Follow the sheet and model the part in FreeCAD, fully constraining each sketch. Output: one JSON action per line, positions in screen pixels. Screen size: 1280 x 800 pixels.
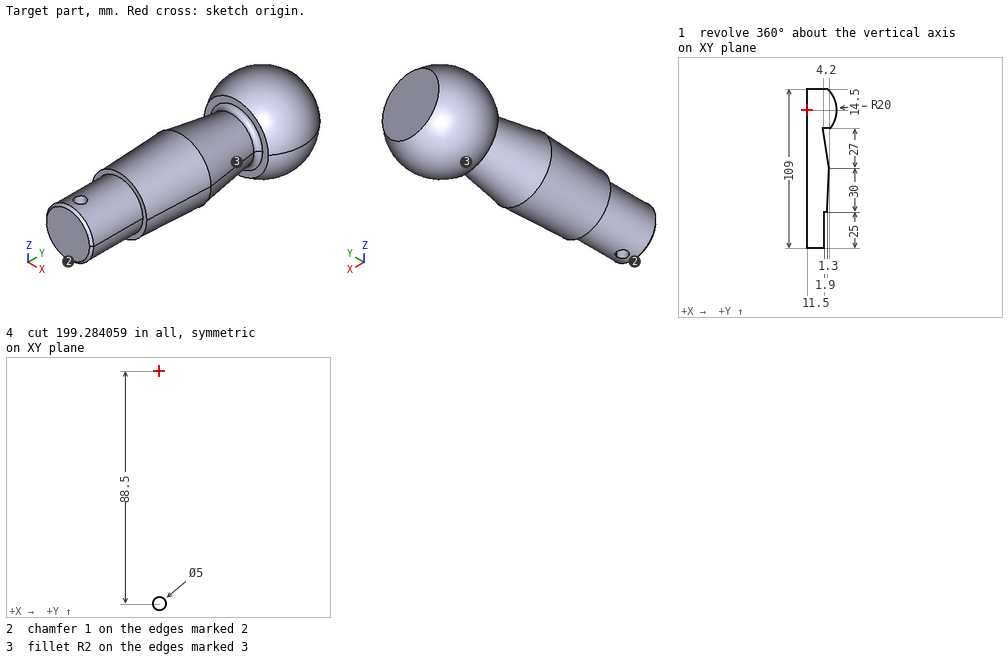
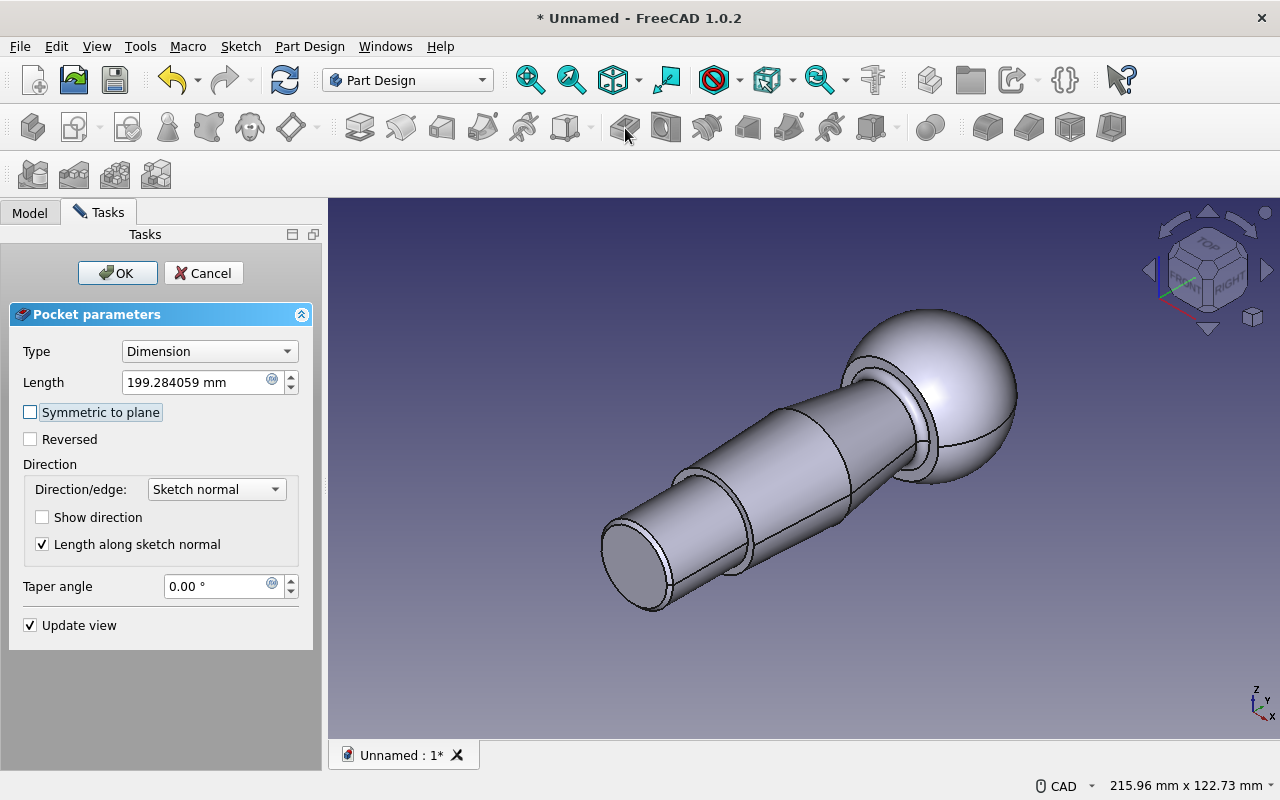
{"action": "left_click", "coordinate": [31, 412]}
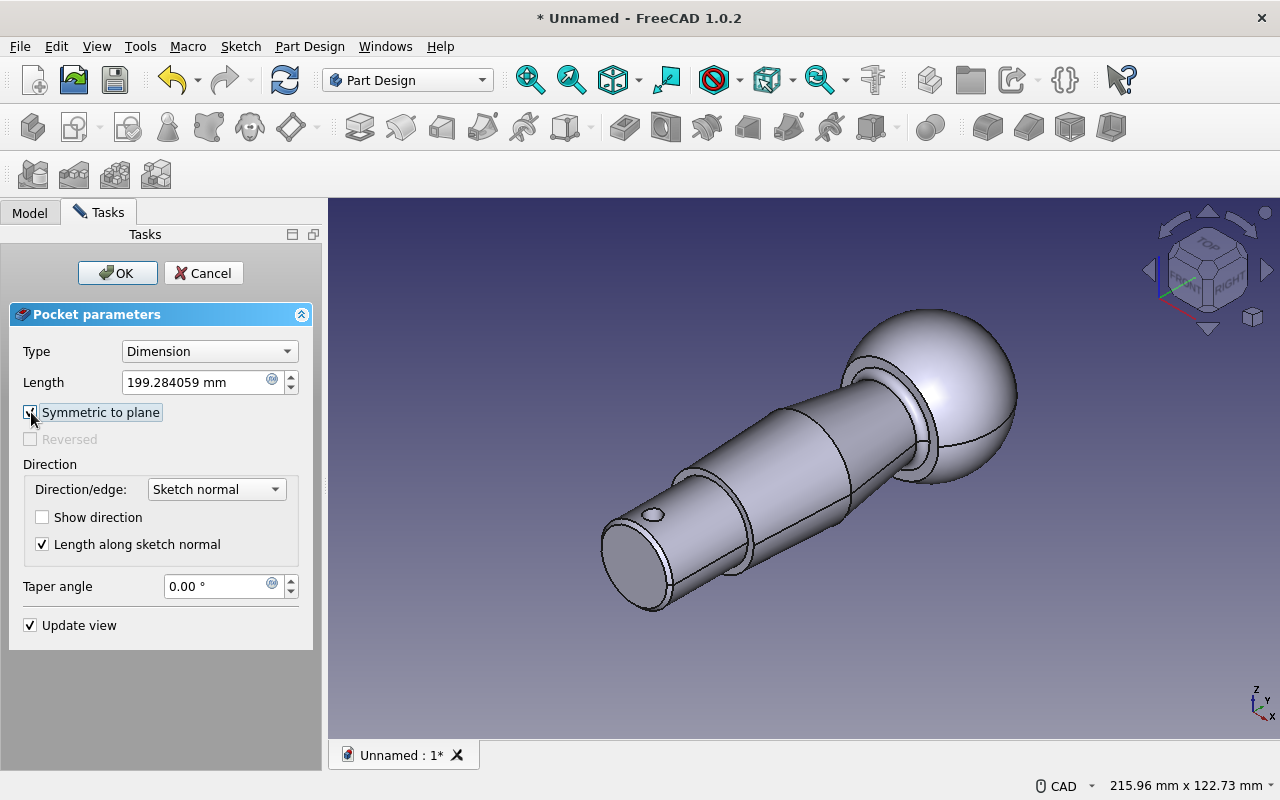
{"action": "left_click", "coordinate": [118, 273]}